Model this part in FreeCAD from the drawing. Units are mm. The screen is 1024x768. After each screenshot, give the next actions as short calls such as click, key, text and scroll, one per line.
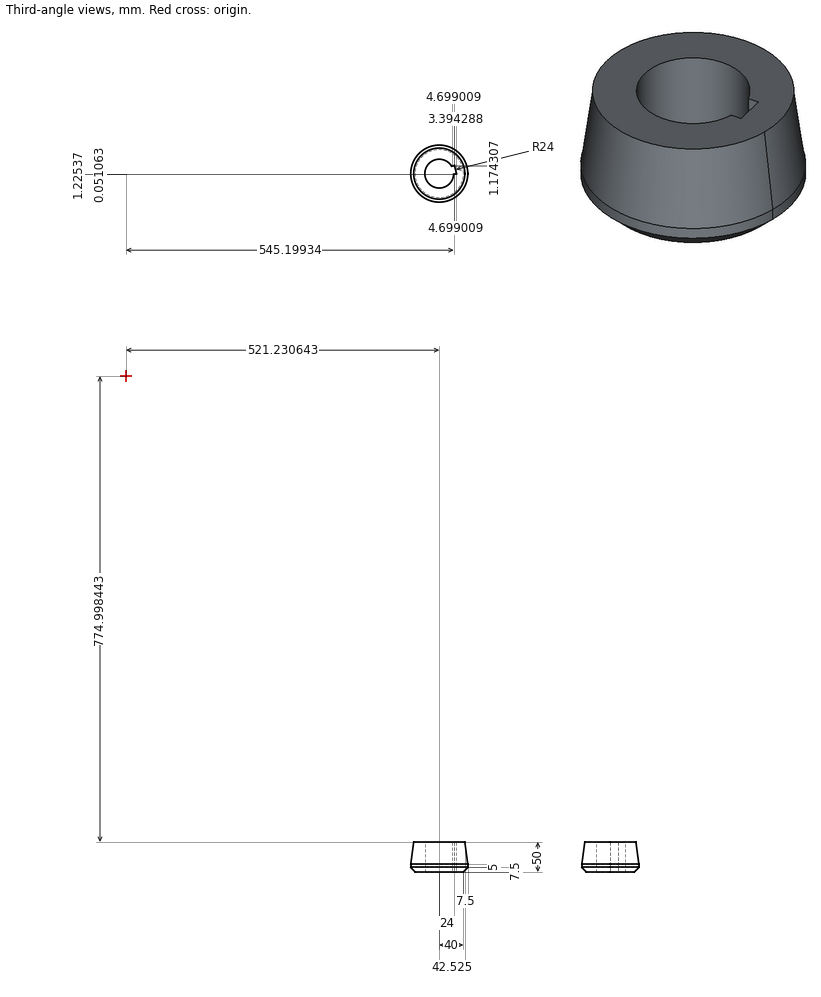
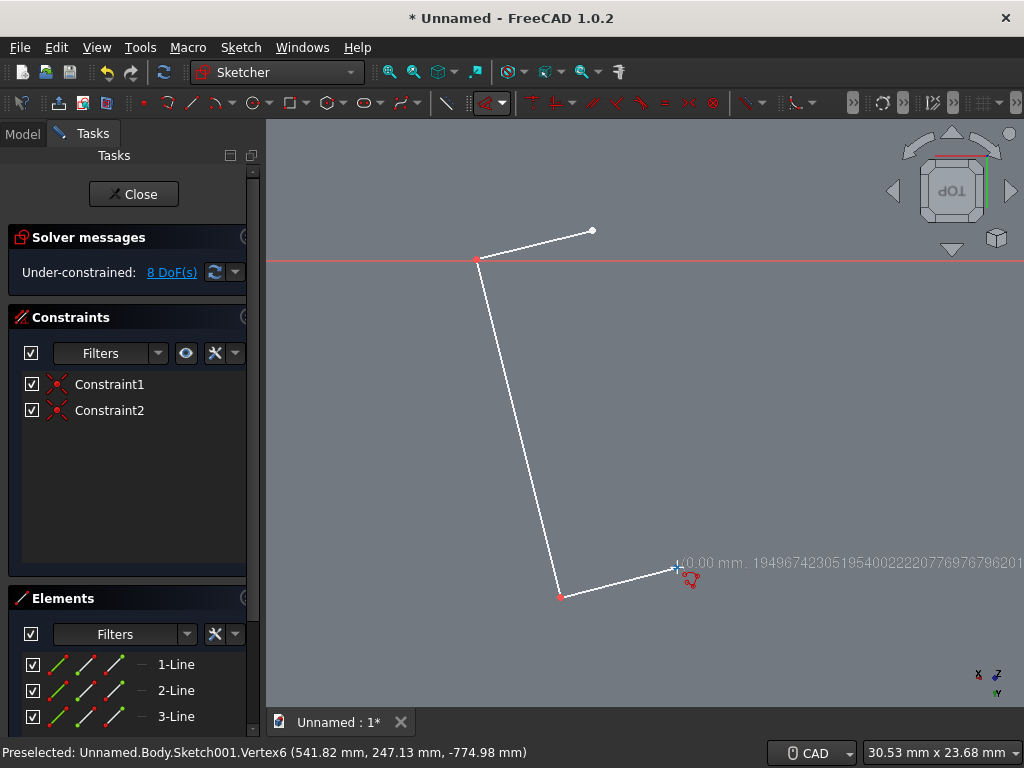
key(g)
key(3)
key(a)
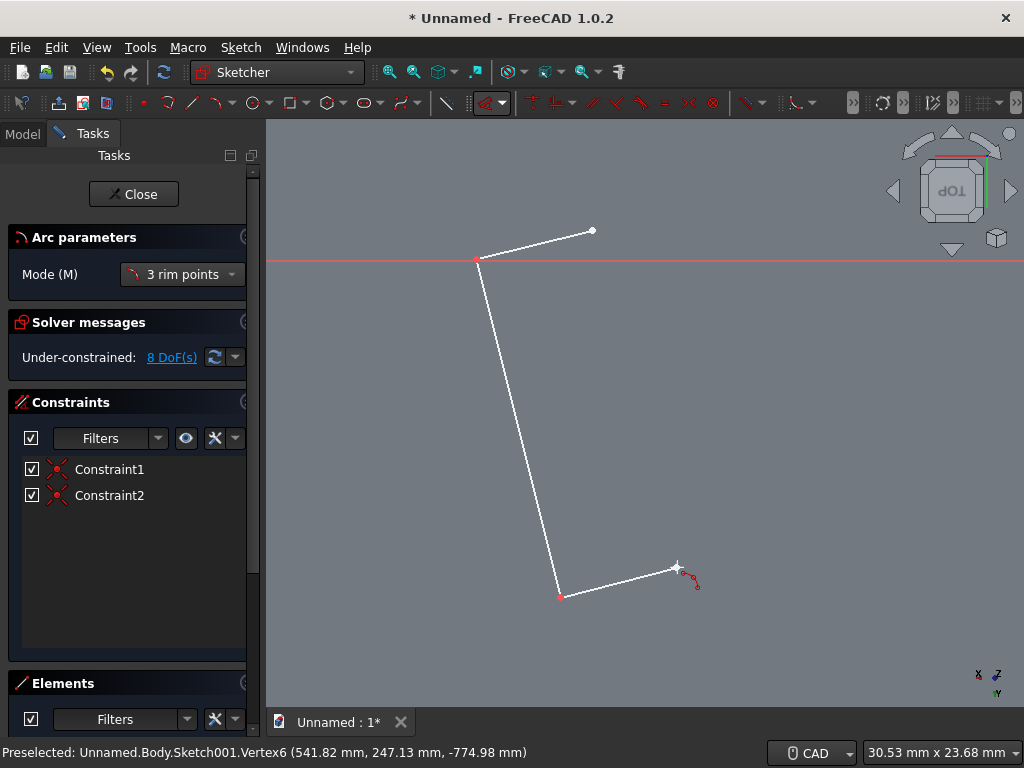
click(677, 568)
click(593, 231)
click(610, 405)
key(Escape)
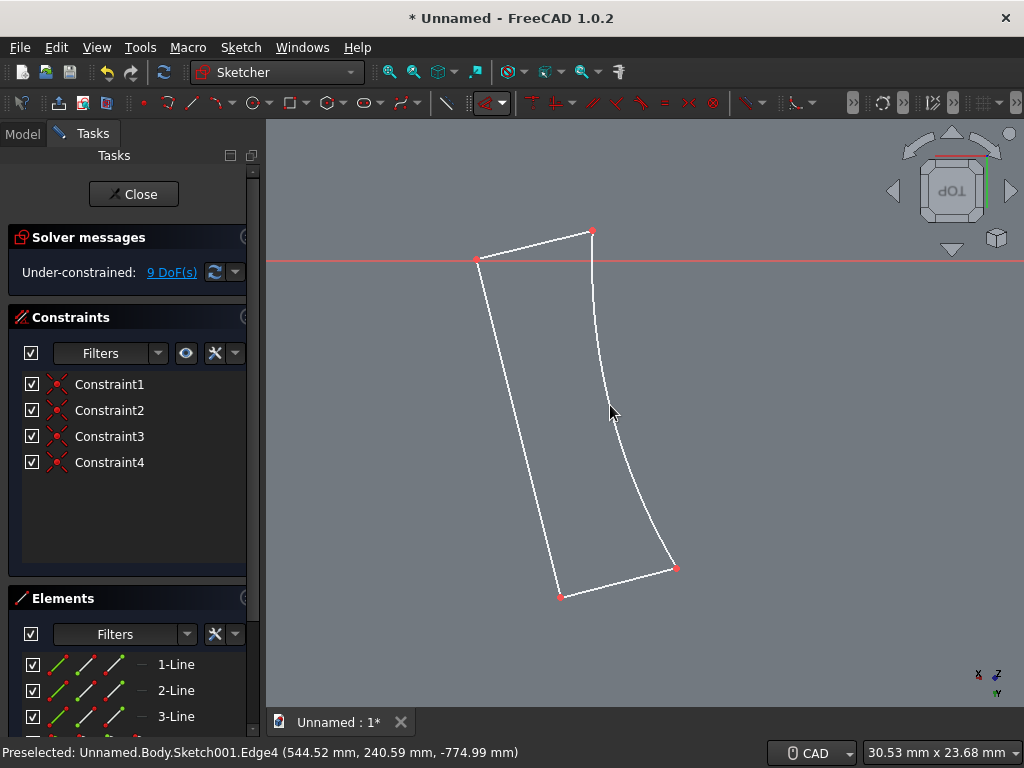
scroll(294, 413, down, 3)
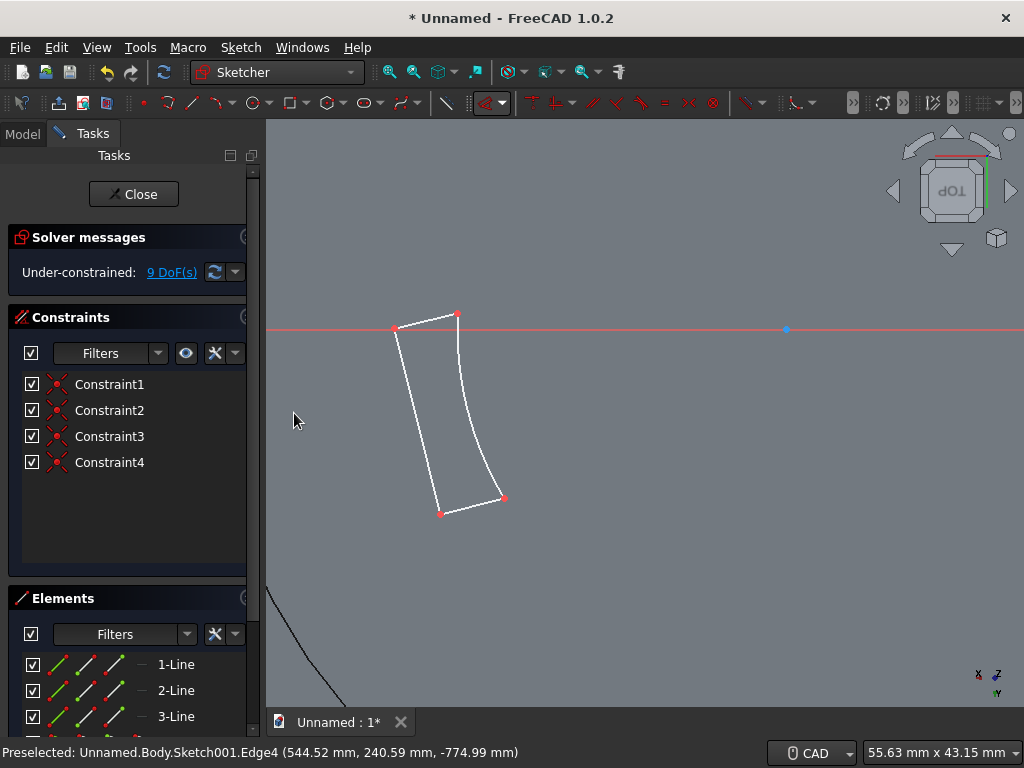
click(787, 329)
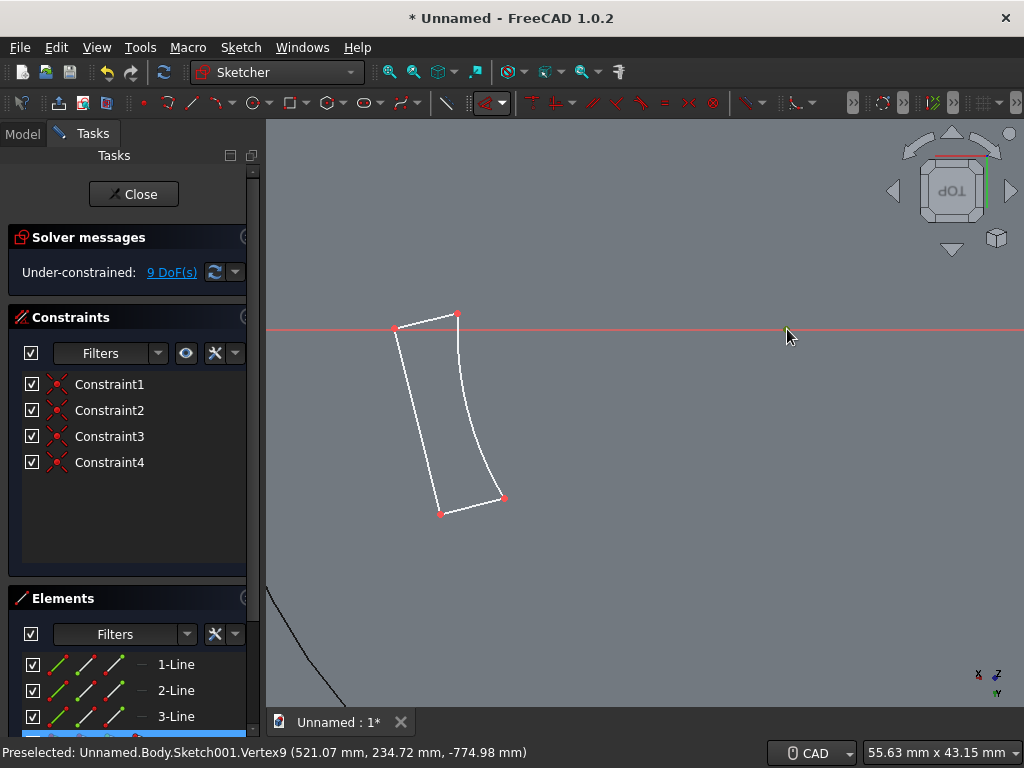
click(334, 330)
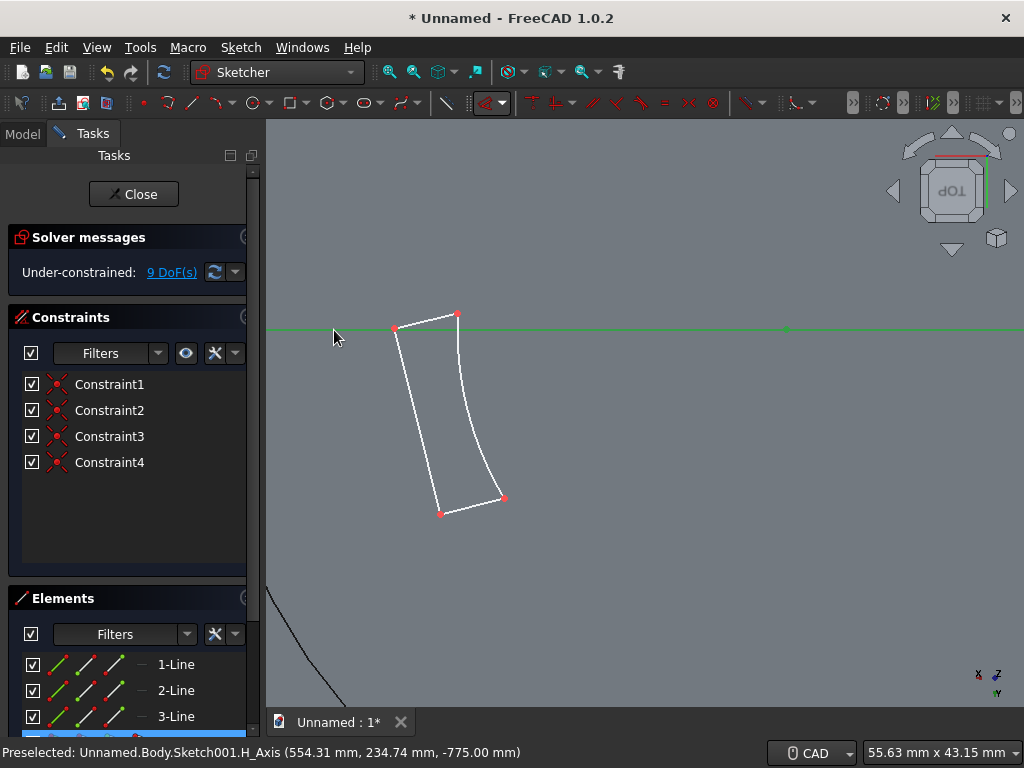
click(532, 104)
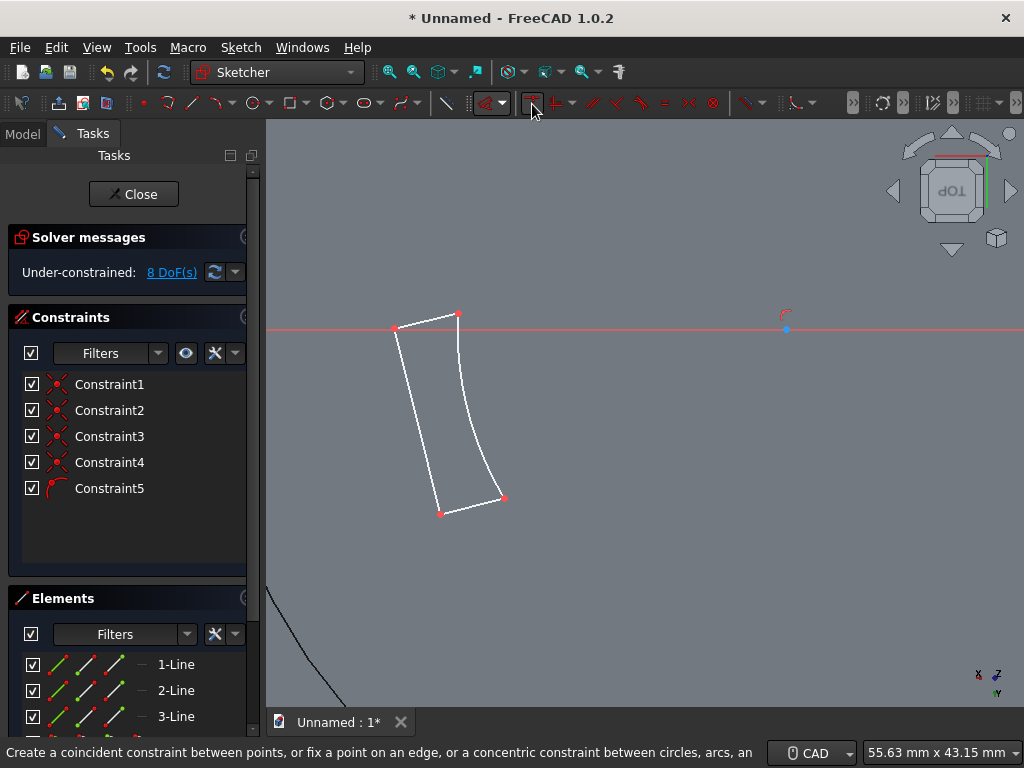
click(460, 371)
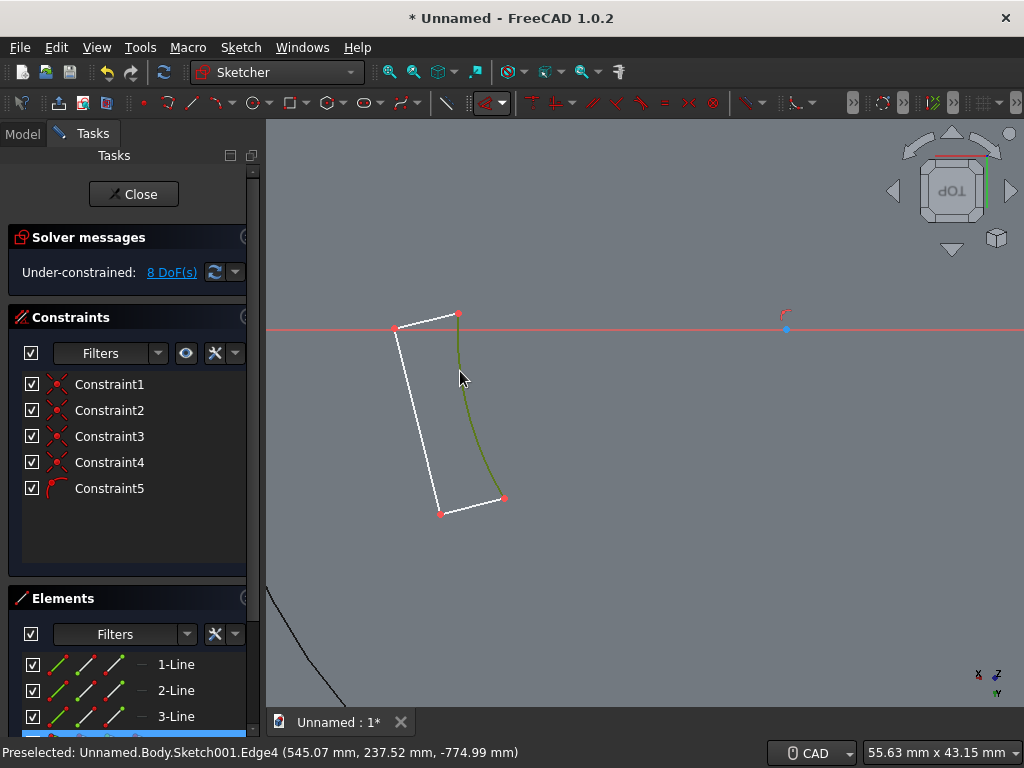
key(k)
key(r)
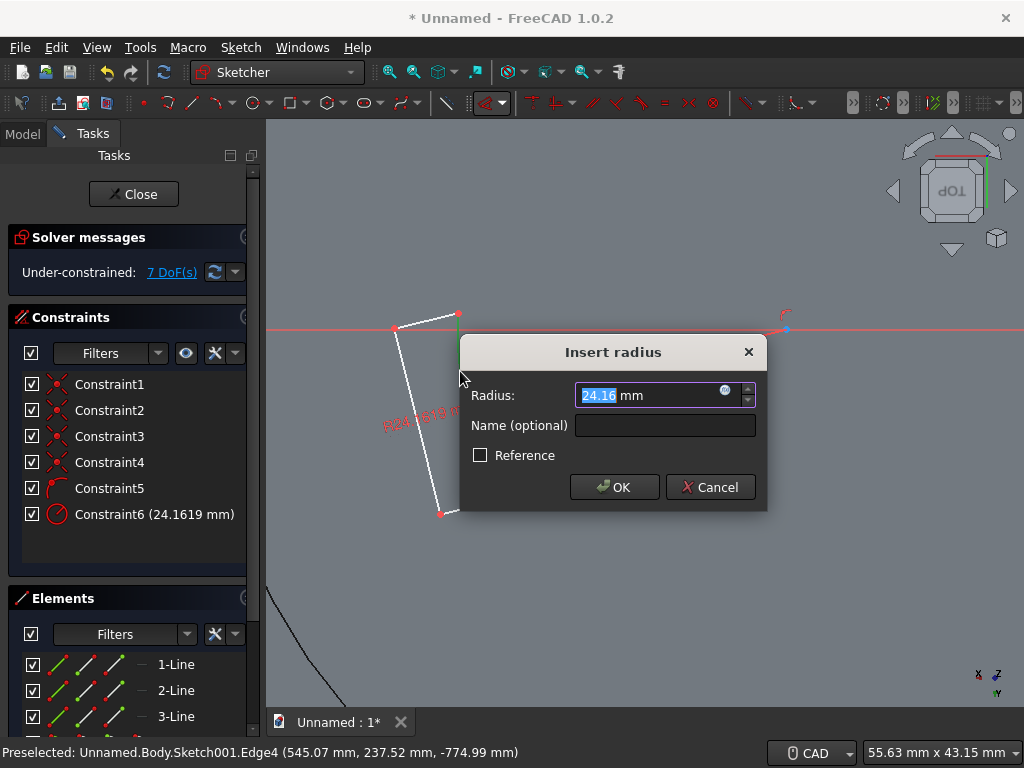
text(24)
key(Return)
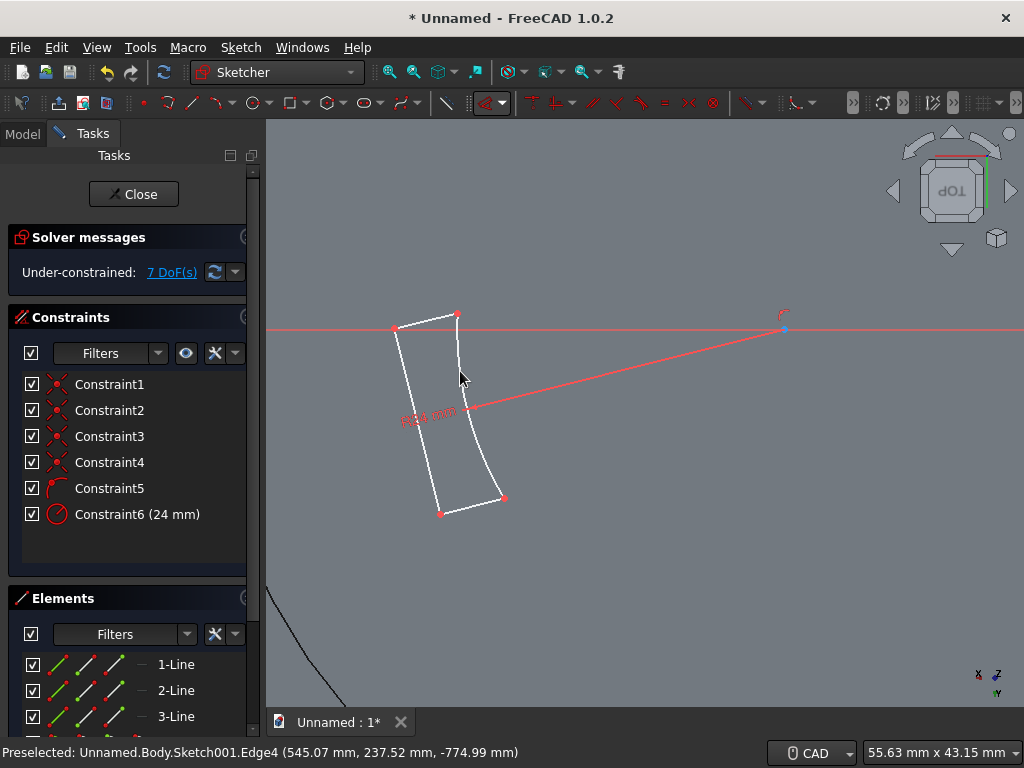
scroll(458, 313, up, 5)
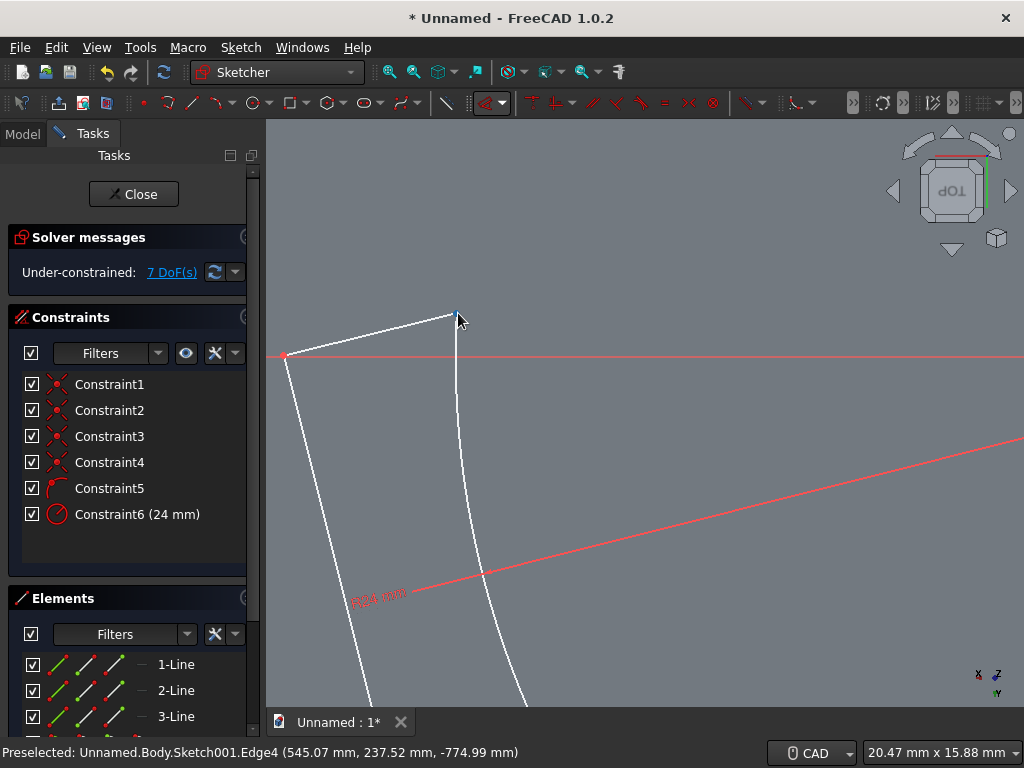
click(457, 313)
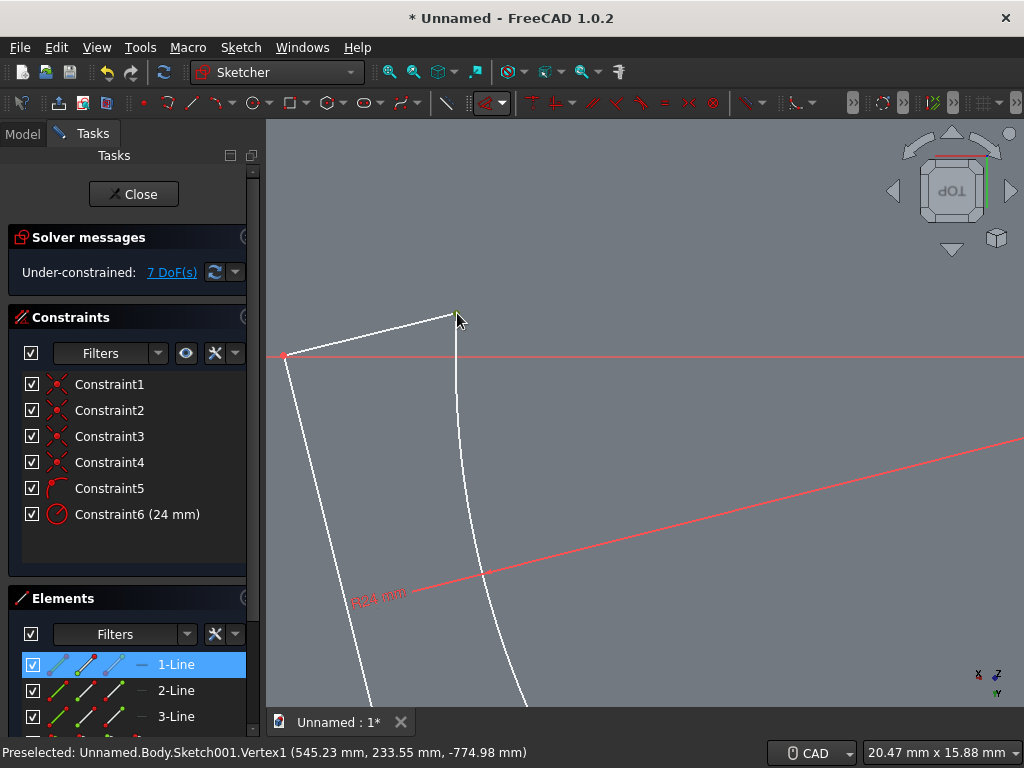
click(504, 104)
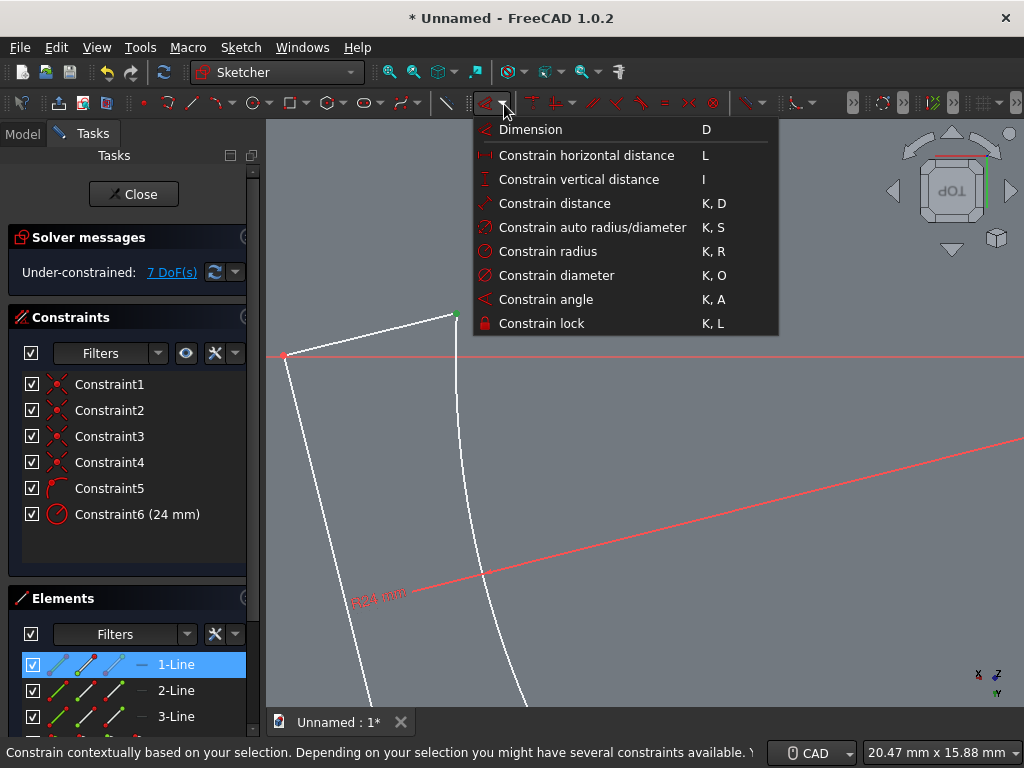
click(626, 179)